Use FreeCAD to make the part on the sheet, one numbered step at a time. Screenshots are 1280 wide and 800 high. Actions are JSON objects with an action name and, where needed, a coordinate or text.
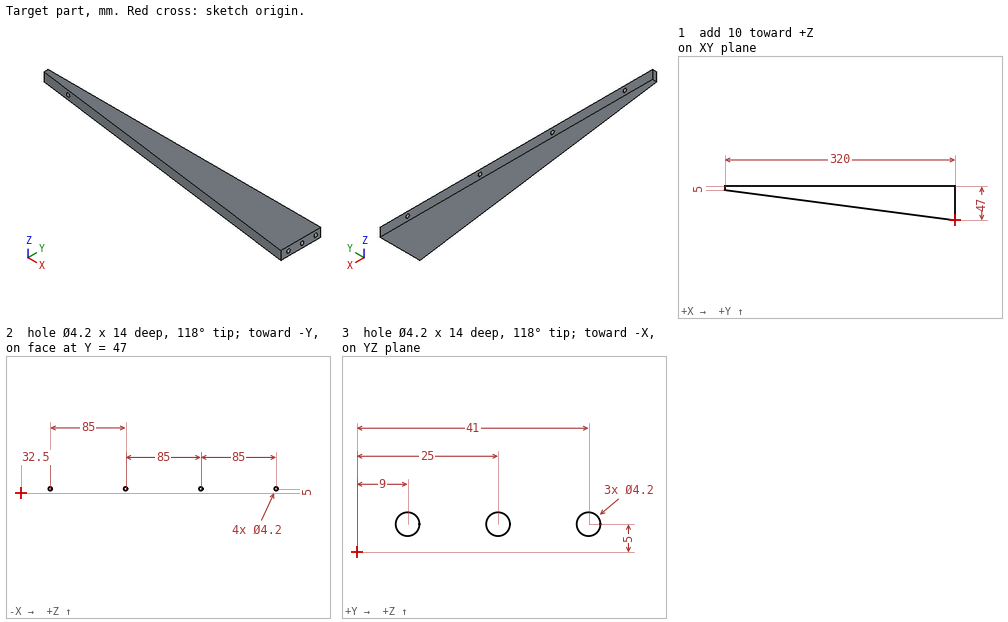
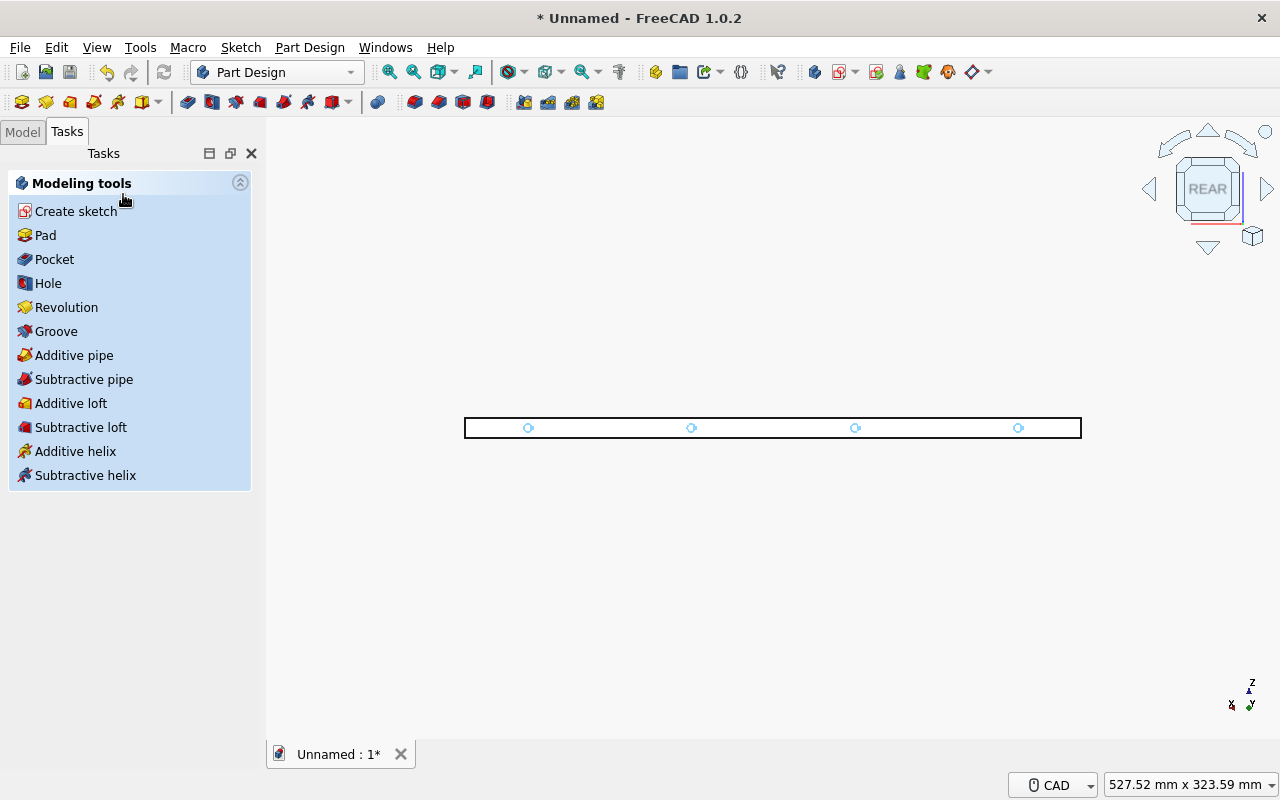
{"action": "left_click", "coordinate": [212, 102]}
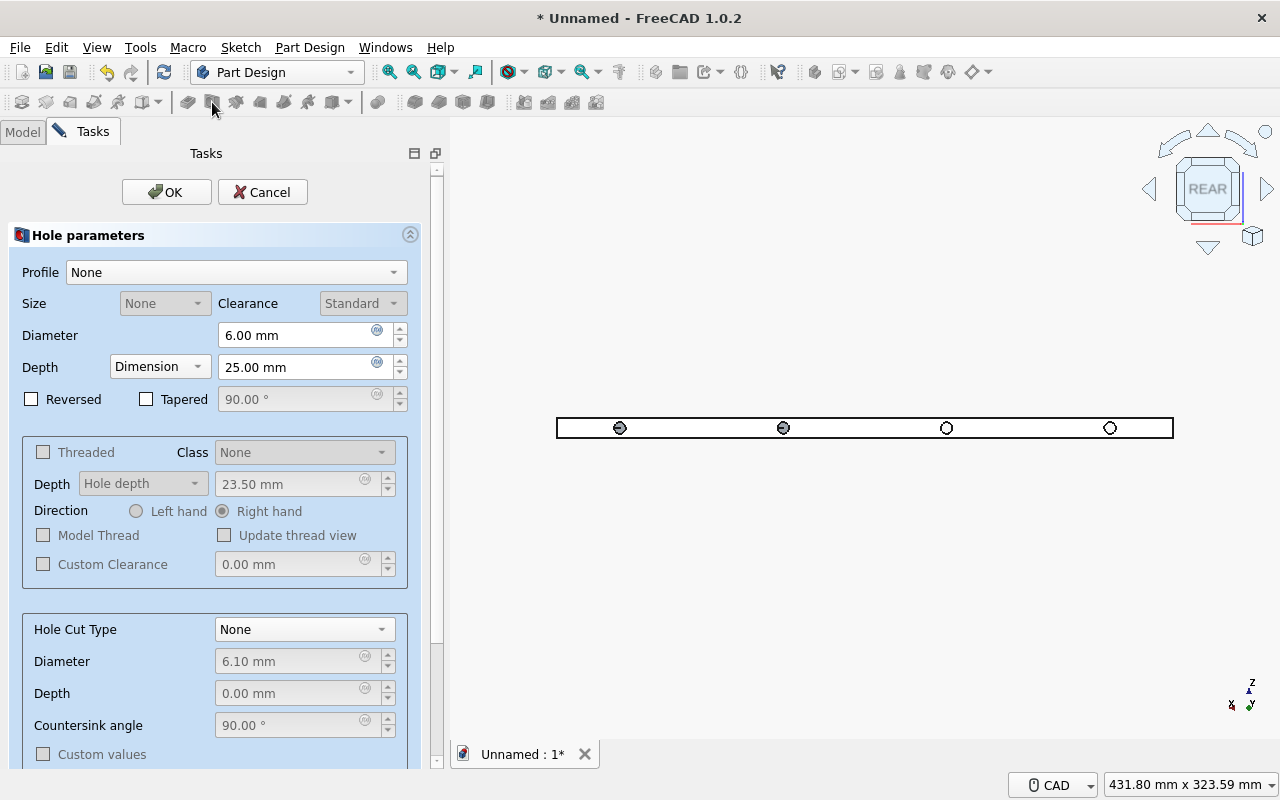
{"action": "triple_click", "coordinate": [305, 335]}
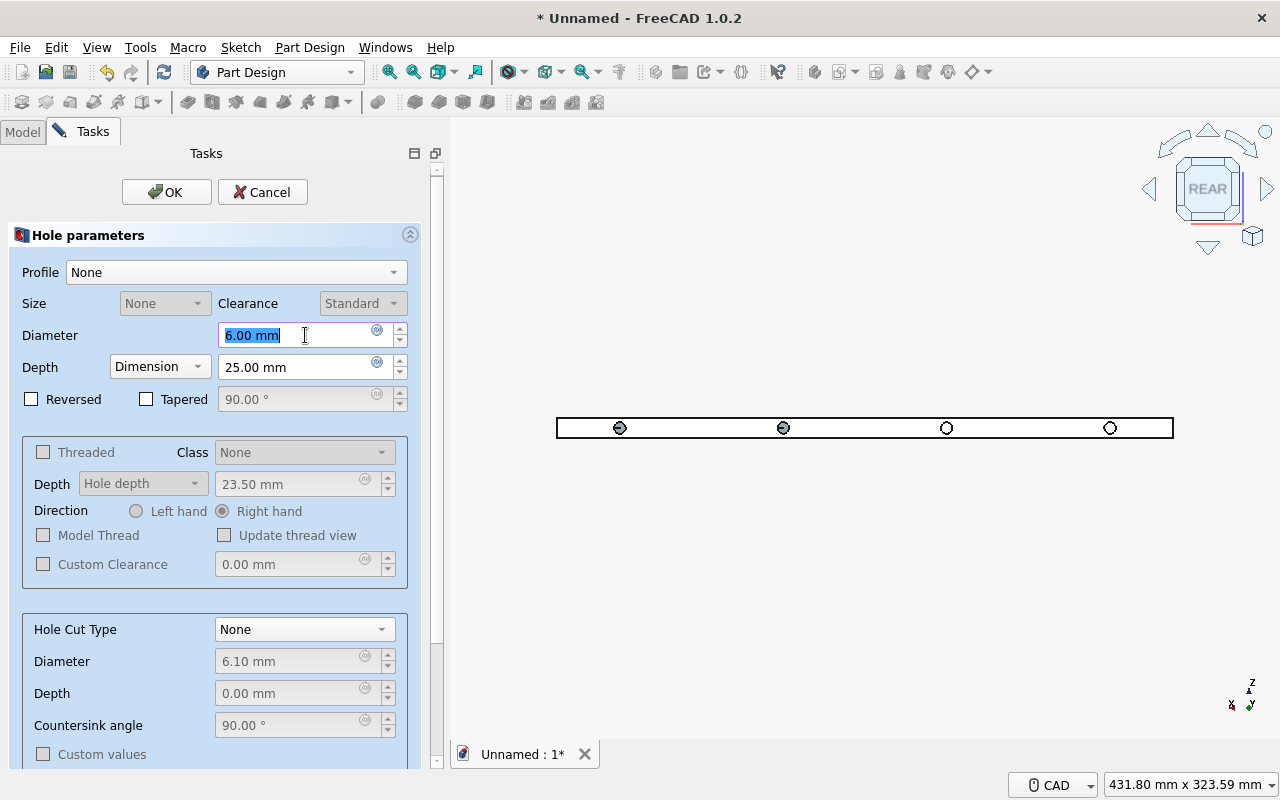
{"action": "type", "text": "4.2"}
{"action": "key", "text": "Tab"}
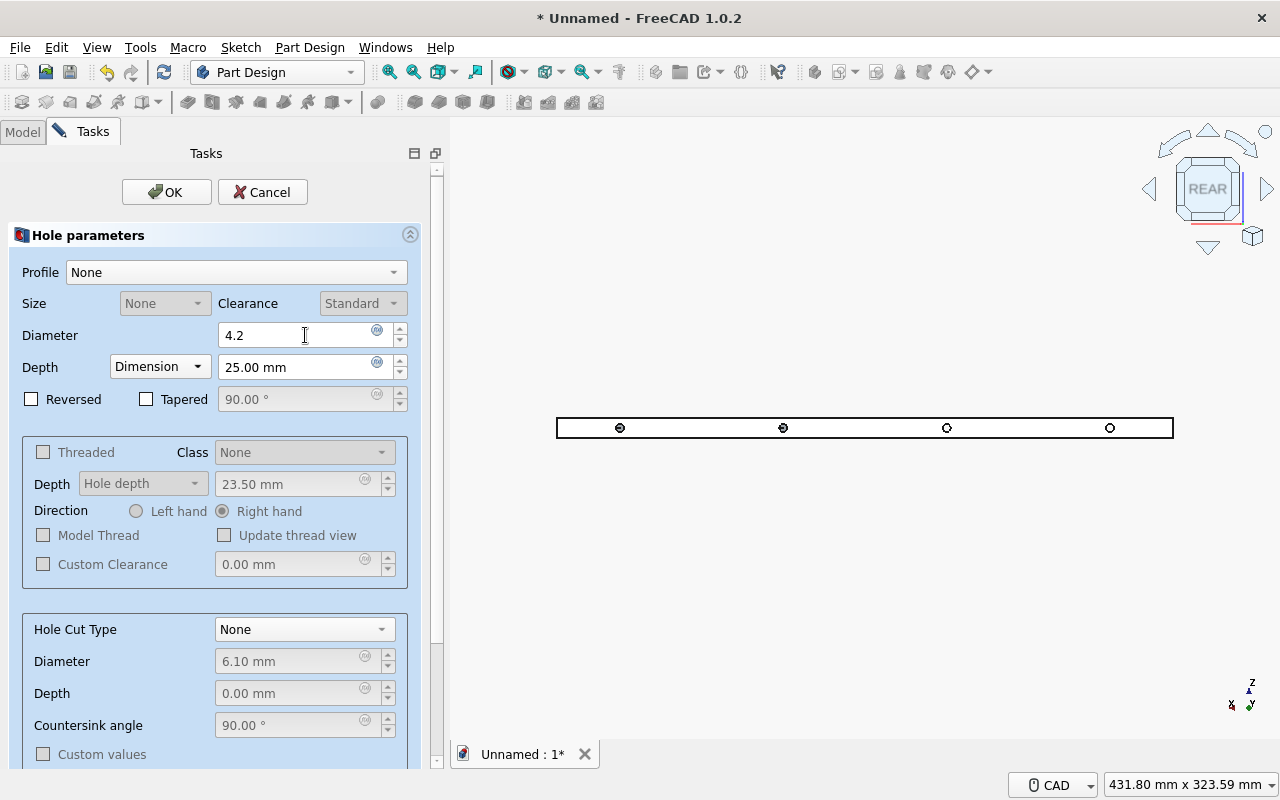
{"action": "triple_click", "coordinate": [305, 367]}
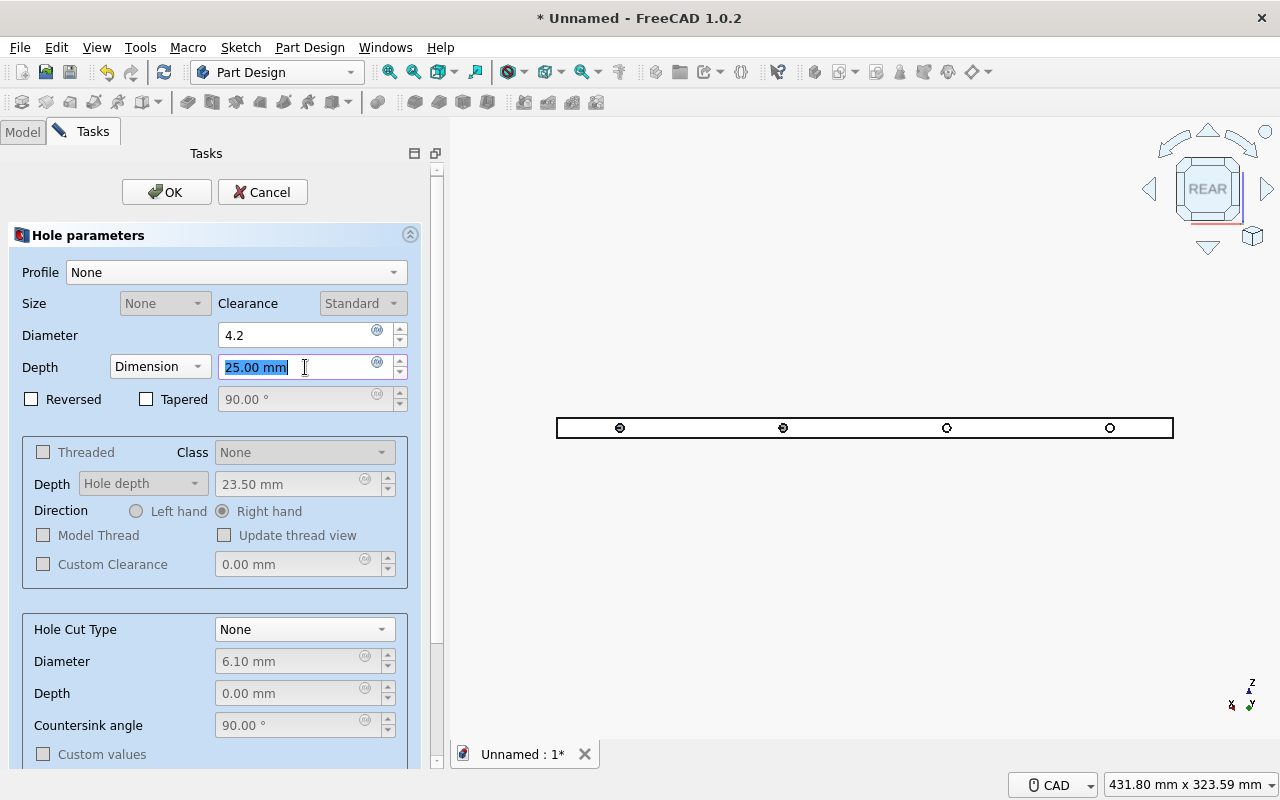
{"action": "type", "text": "14"}
{"action": "key", "text": "Tab"}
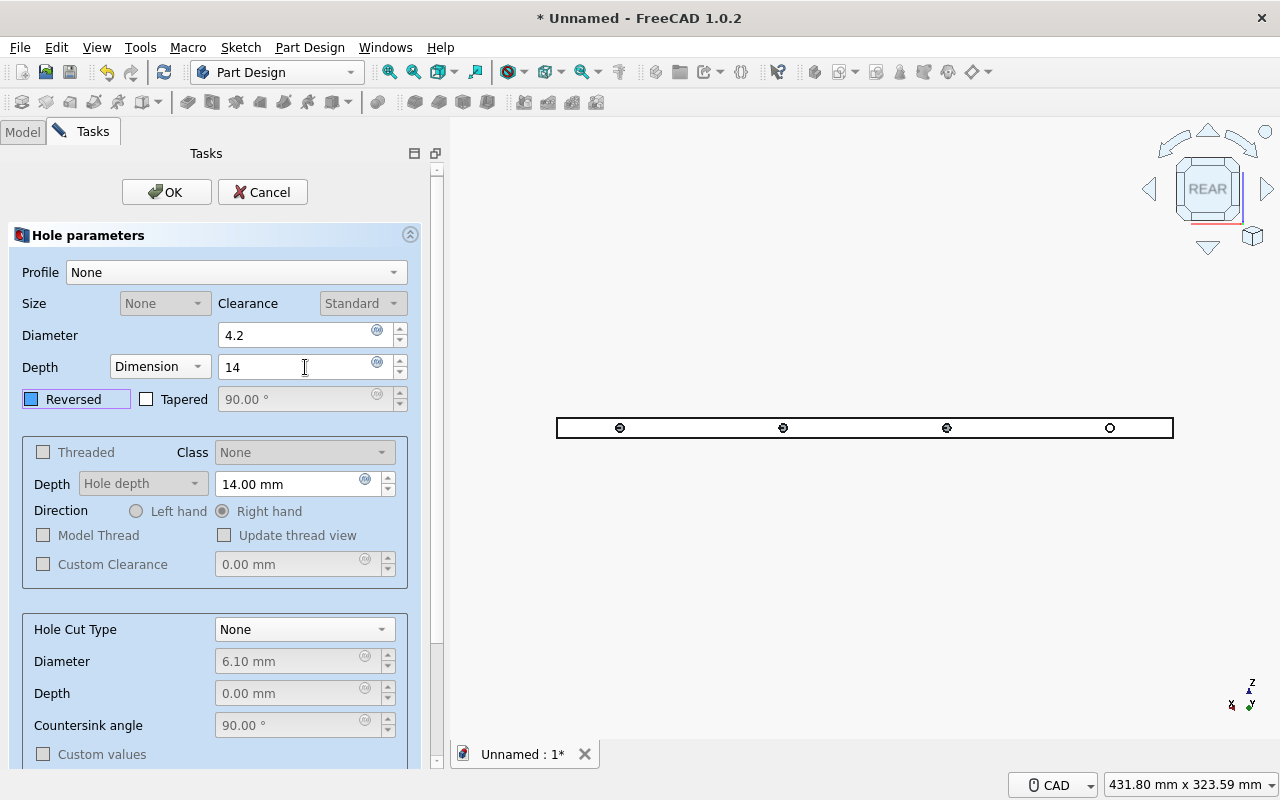
{"action": "left_click", "coordinate": [167, 192]}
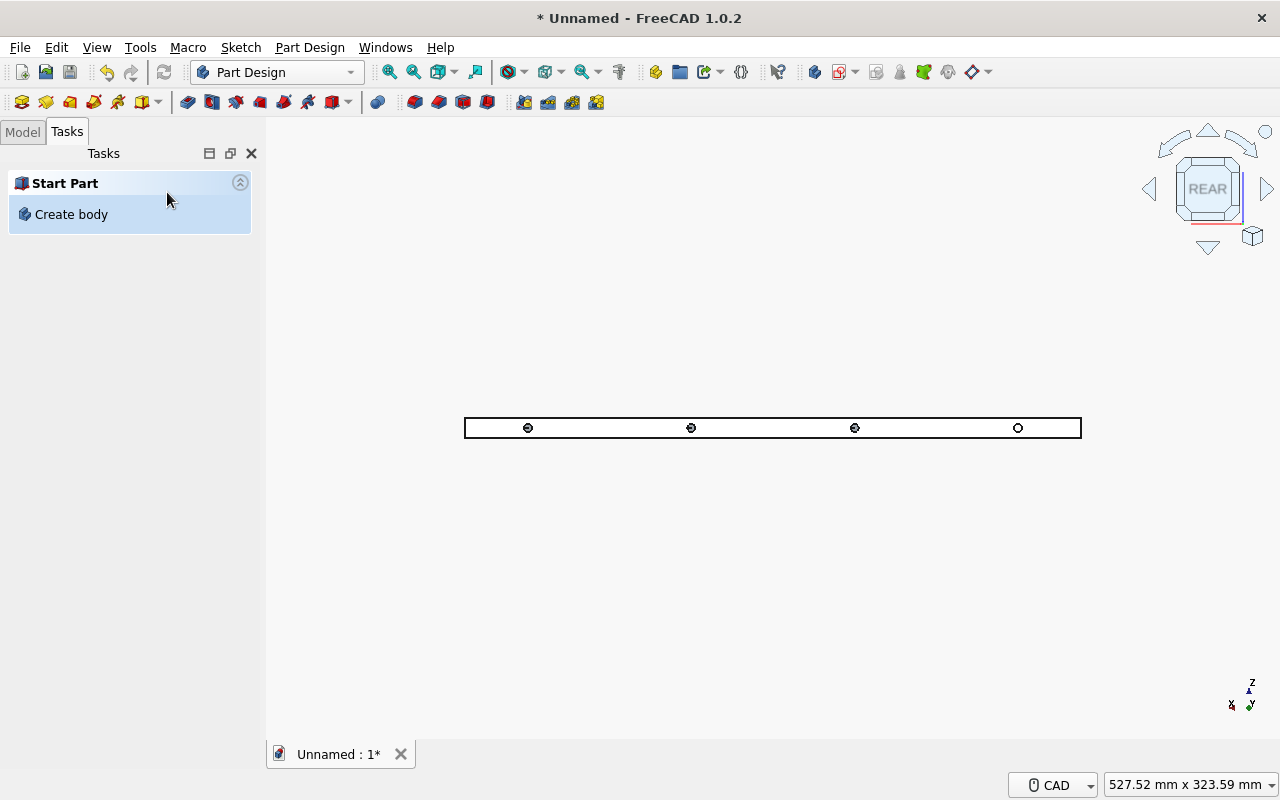
{"action": "left_click", "coordinate": [840, 72]}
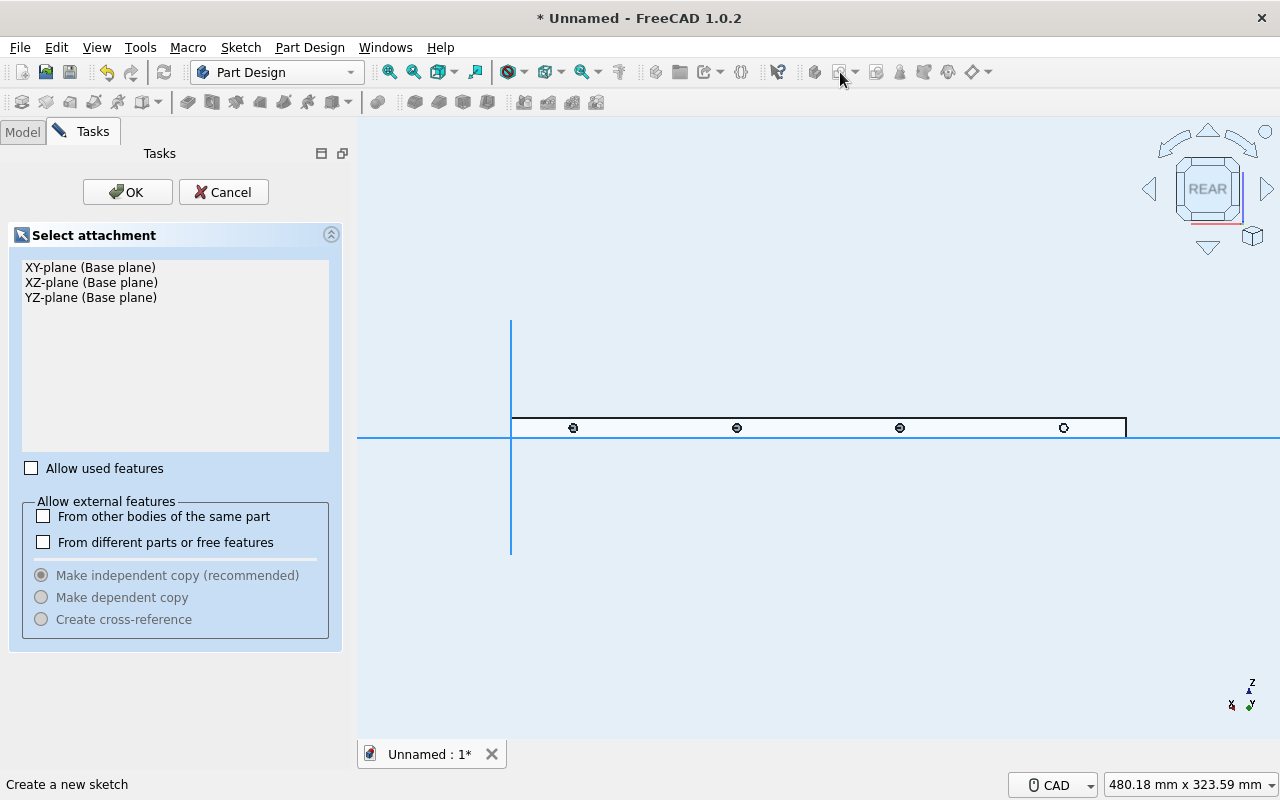
{"action": "left_click", "coordinate": [82, 298]}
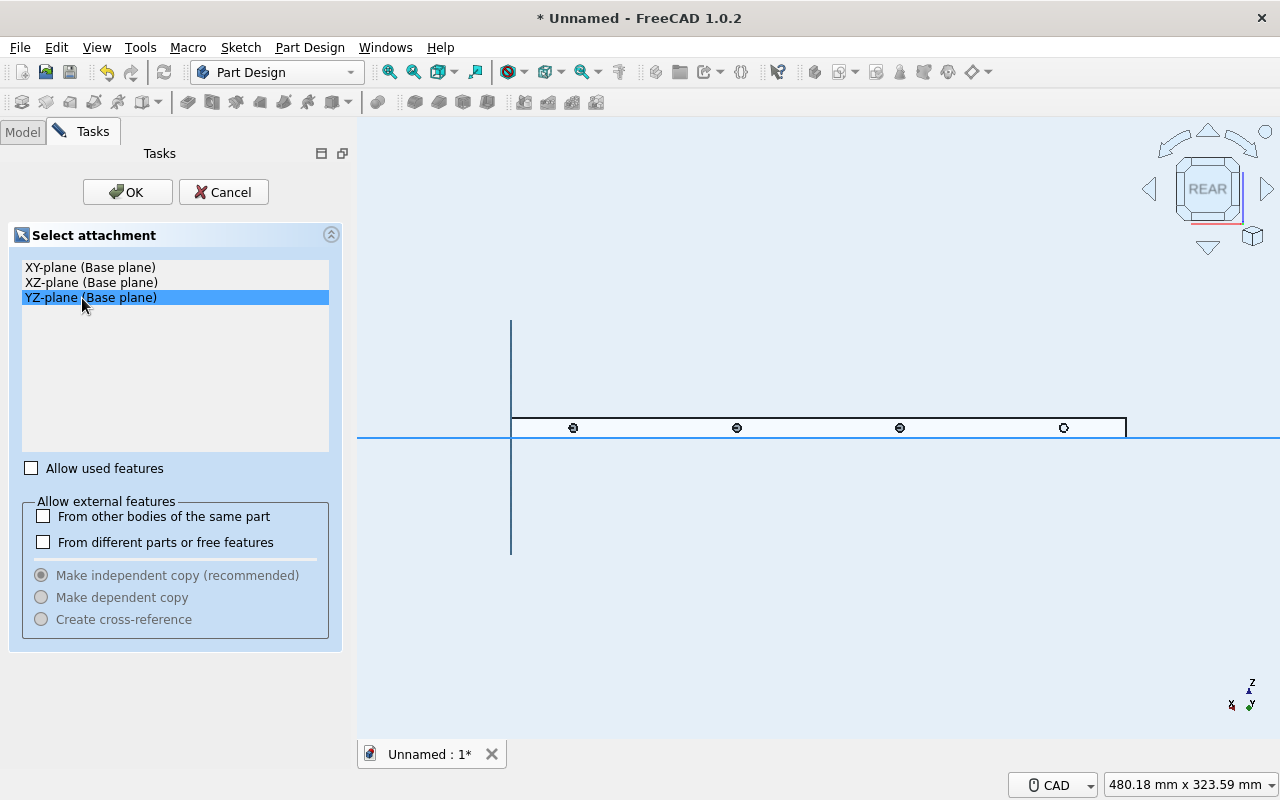
{"action": "left_click", "coordinate": [128, 192]}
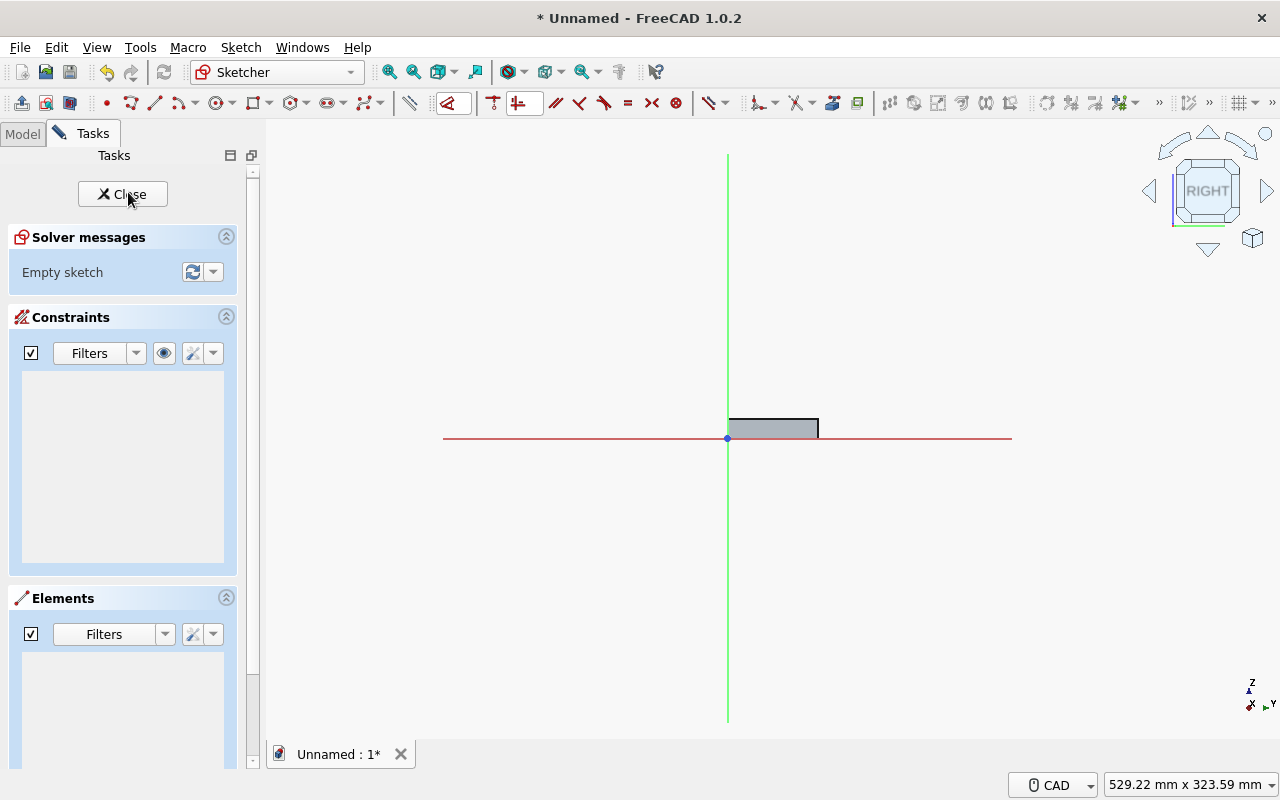
{"action": "scroll", "coordinate": [779, 432], "scroll_direction": "up", "scroll_amount": 10}